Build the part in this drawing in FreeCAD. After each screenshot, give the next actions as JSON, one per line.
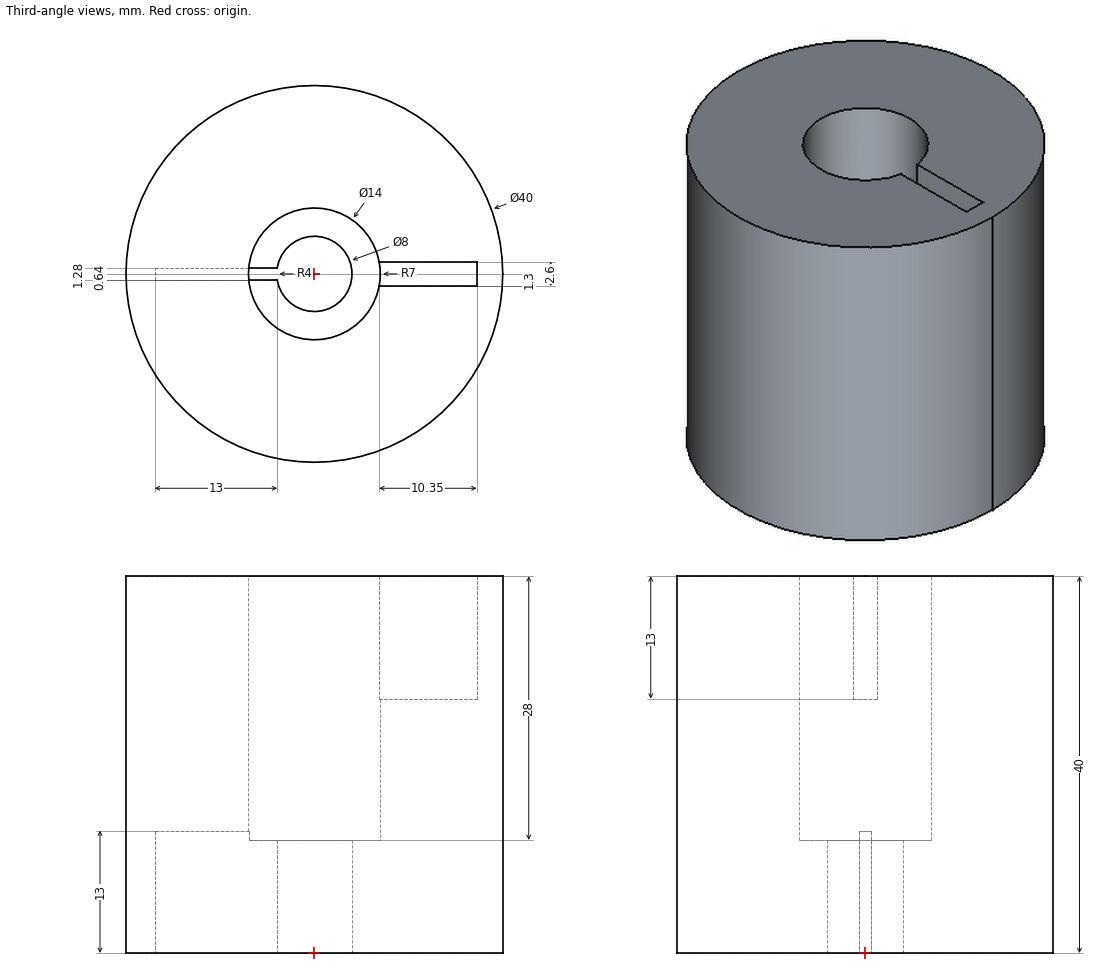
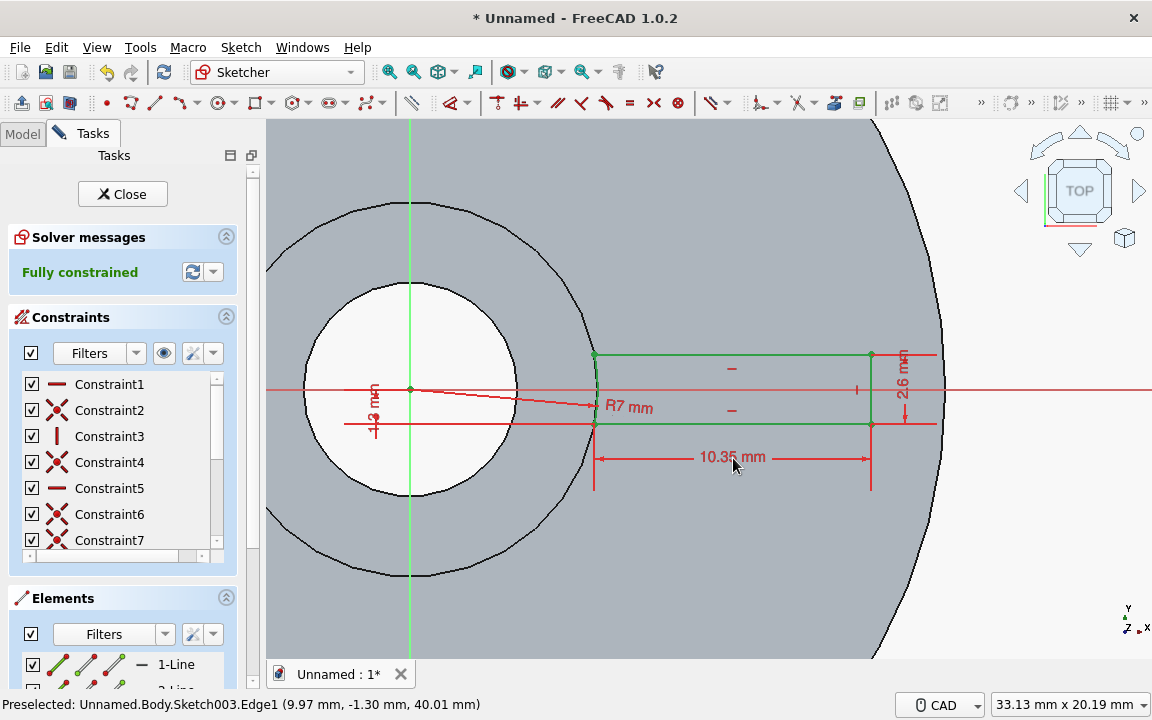
{"action": "left_click", "coordinate": [123, 194]}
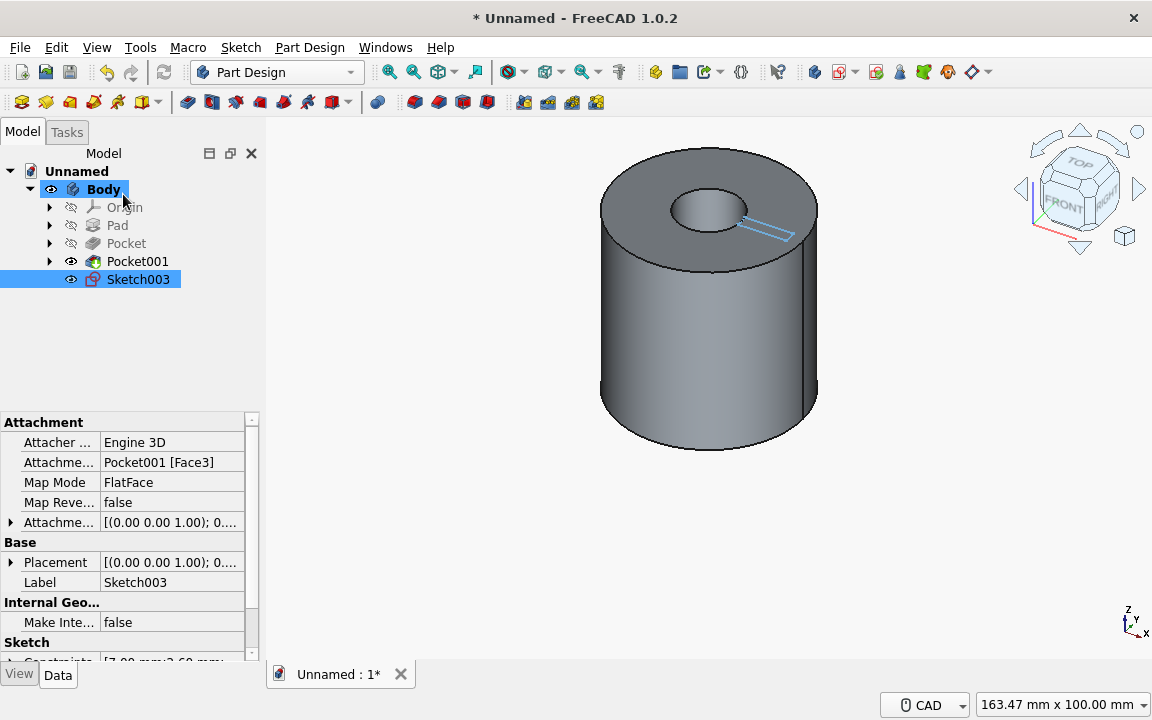
{"action": "left_click", "coordinate": [188, 102]}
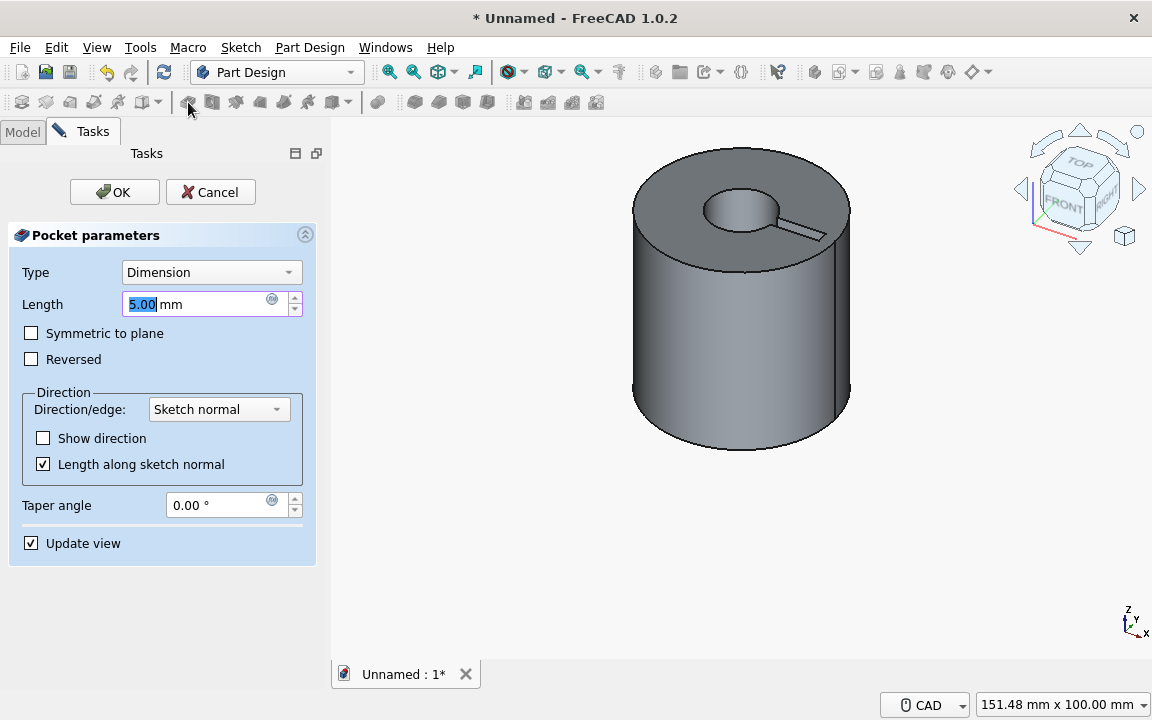
{"action": "type", "text": "13"}
{"action": "key", "text": "Tab"}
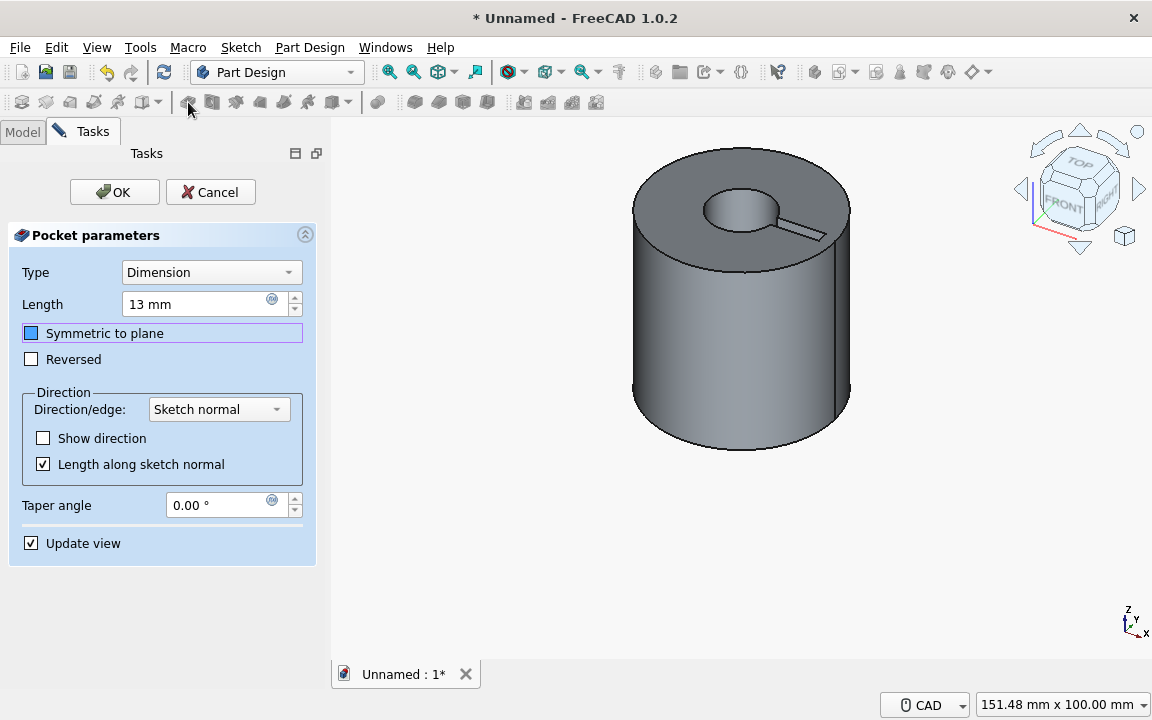
{"action": "left_click", "coordinate": [115, 192]}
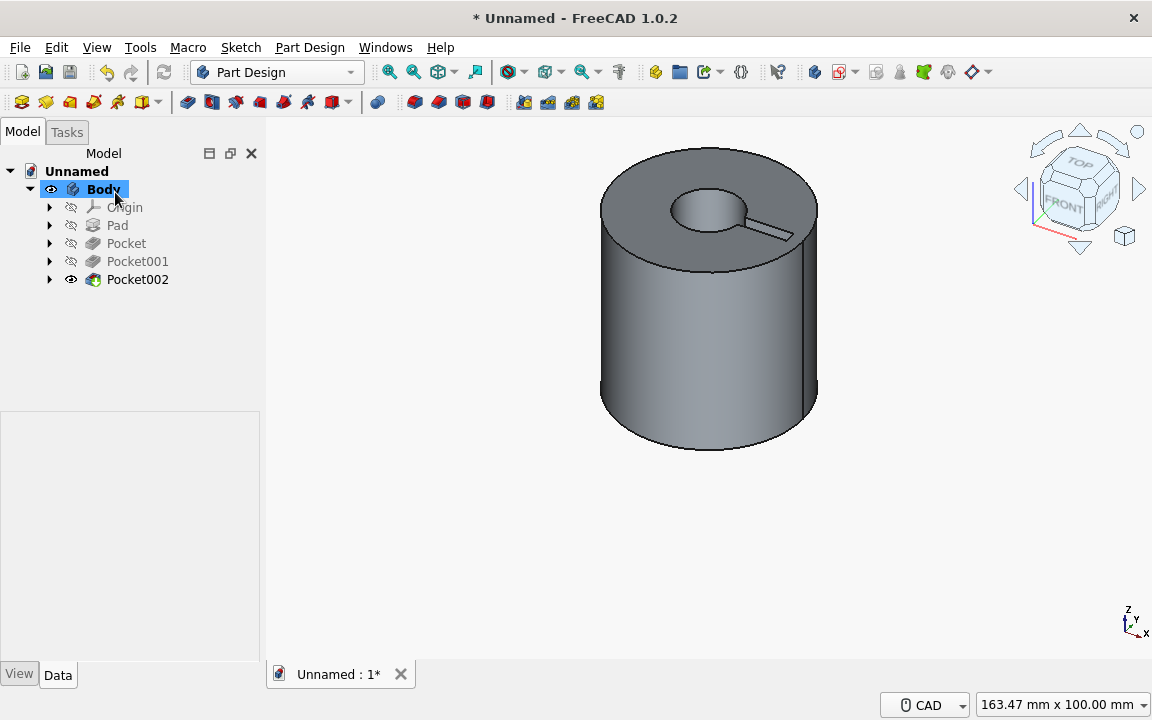
{"action": "left_click", "coordinate": [50, 207]}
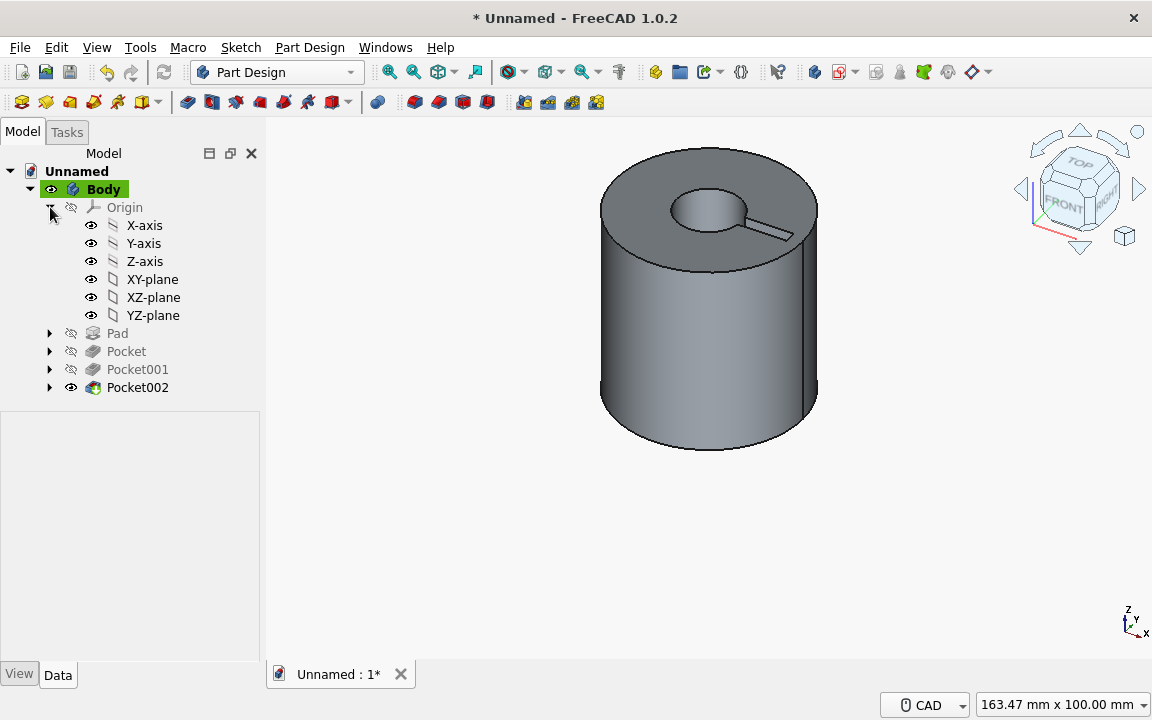
{"action": "left_click", "coordinate": [136, 279]}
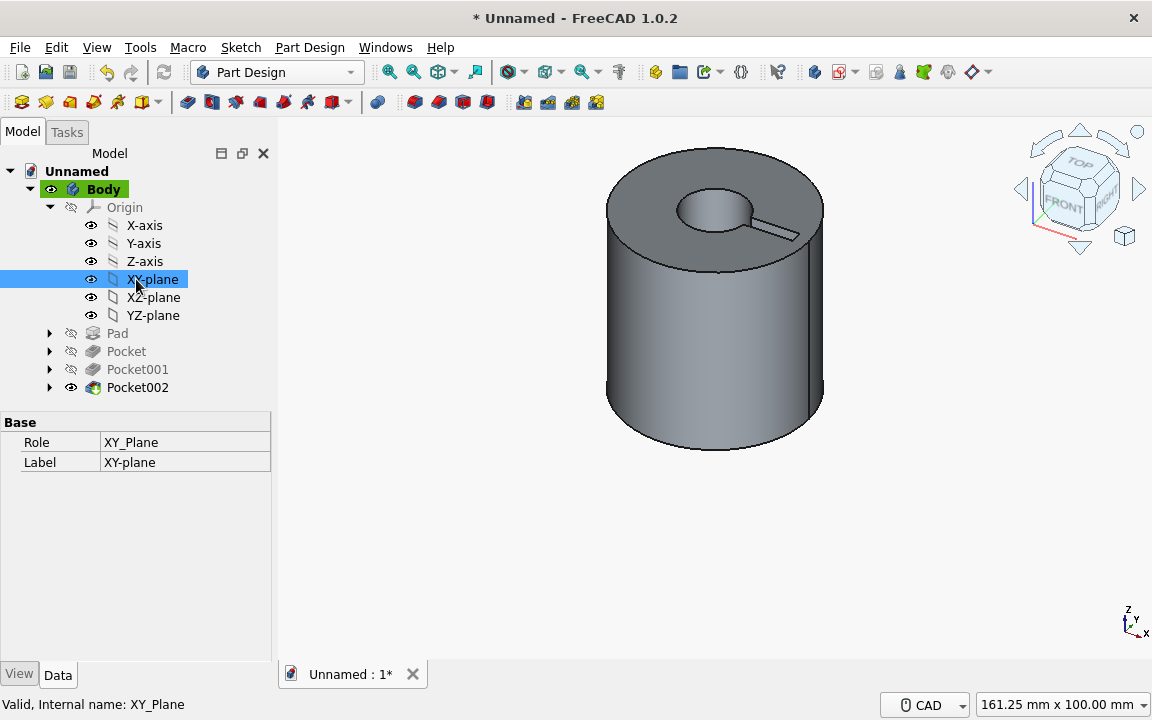
{"action": "left_click", "coordinate": [972, 72]}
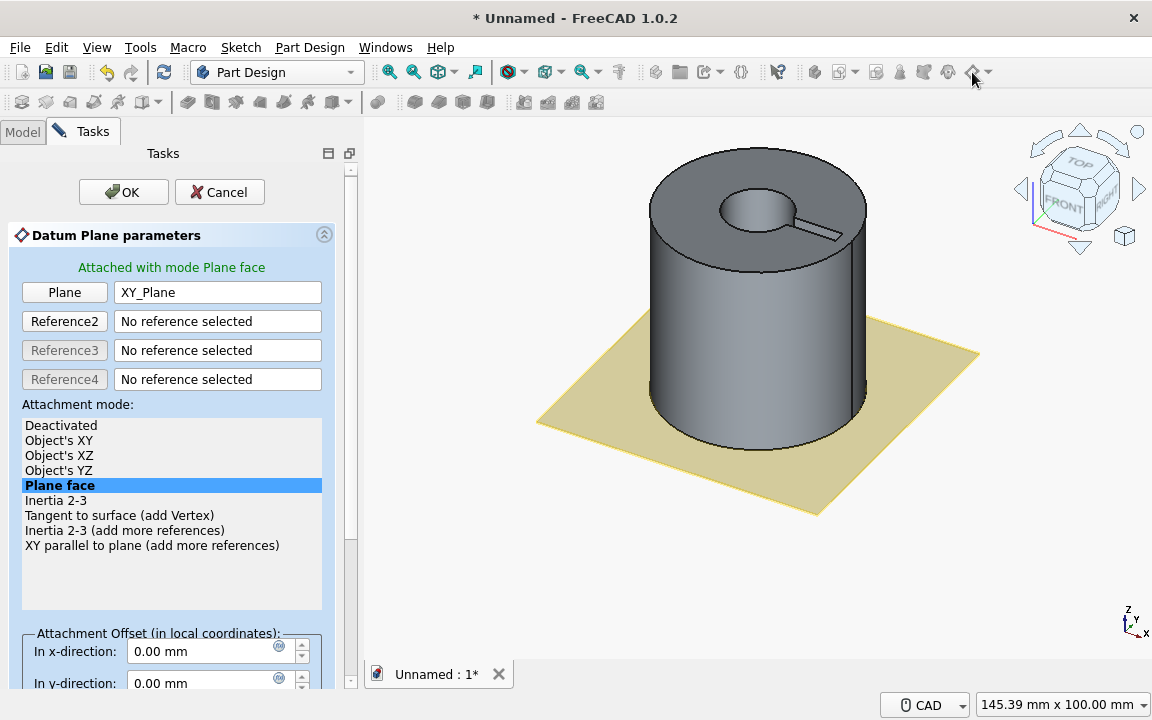
{"action": "scroll", "coordinate": [351, 426], "scroll_direction": "down", "scroll_amount": 2}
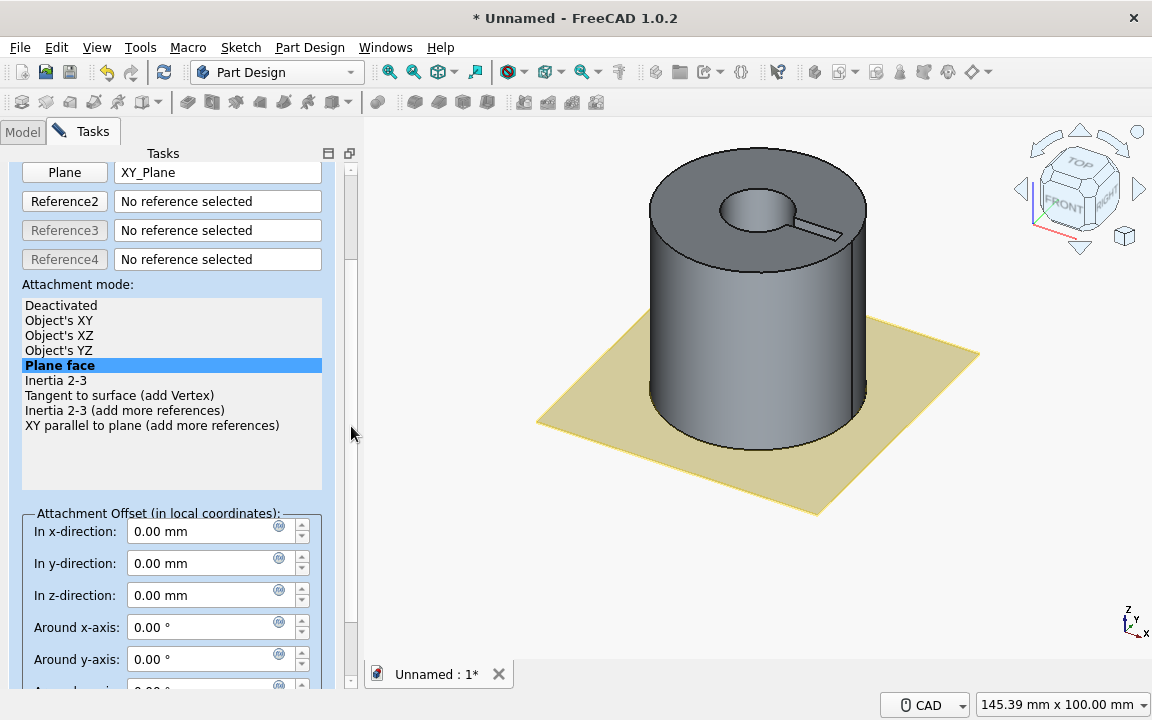
{"action": "triple_click", "coordinate": [210, 595]}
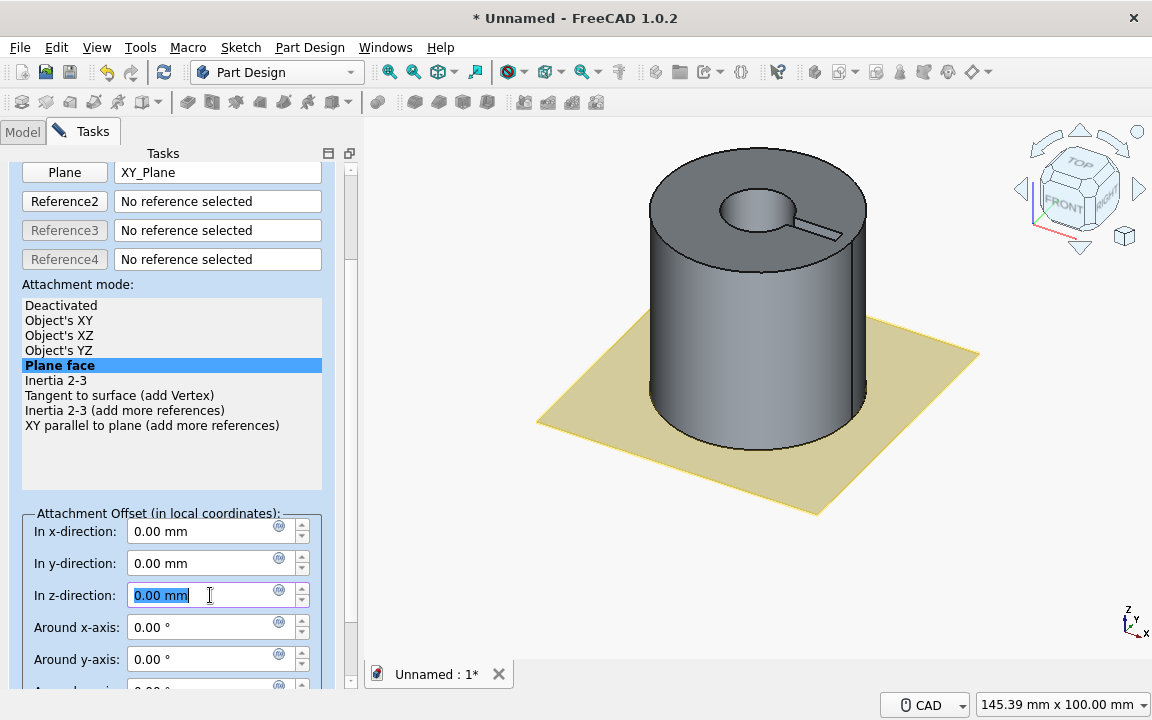
{"action": "type", "text": "13"}
{"action": "key", "text": "Tab"}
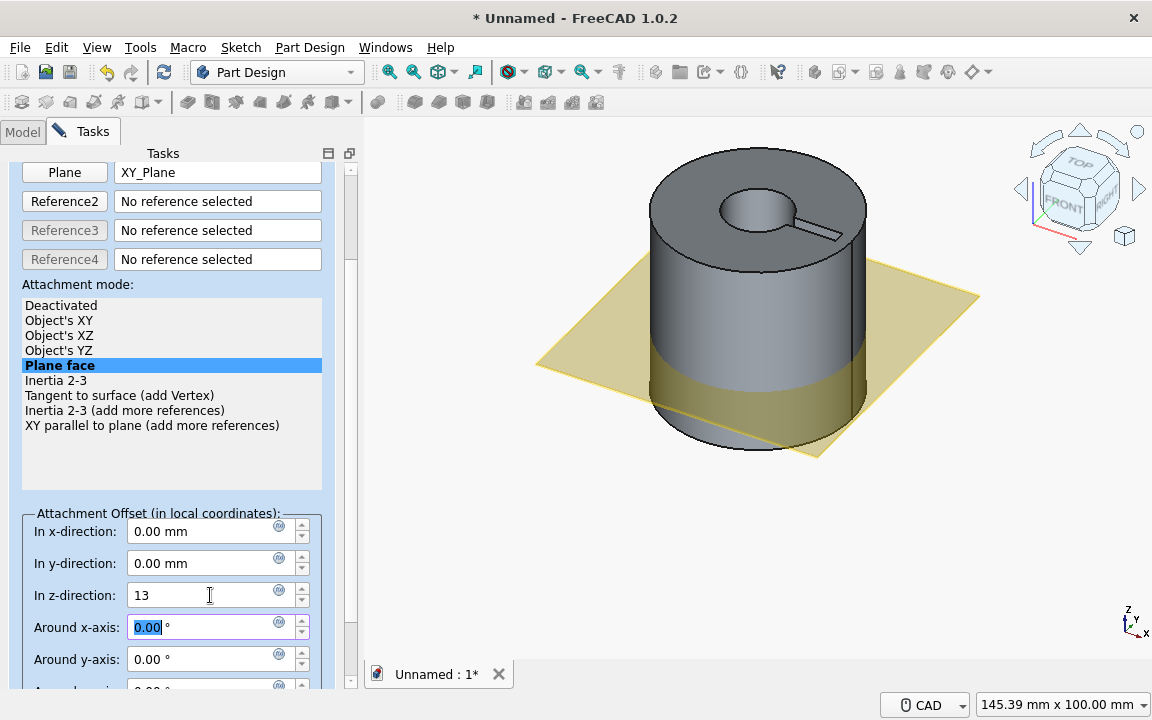
{"action": "scroll", "coordinate": [351, 426], "scroll_direction": "up", "scroll_amount": 3}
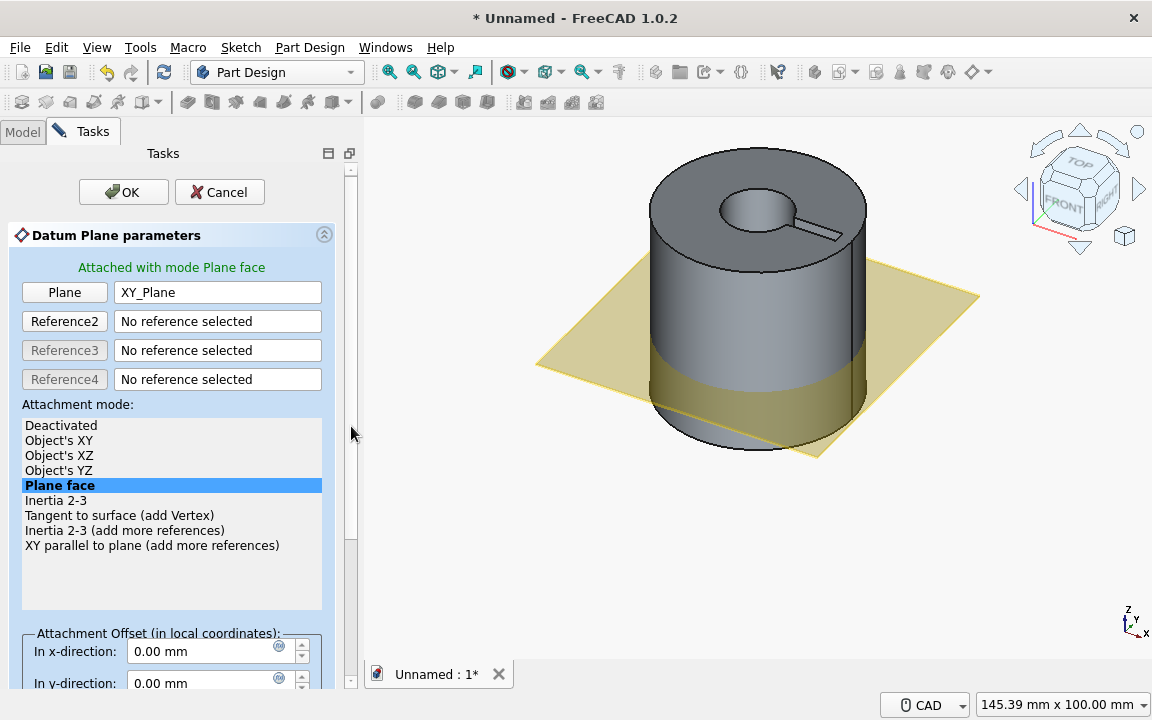
{"action": "left_click", "coordinate": [124, 192]}